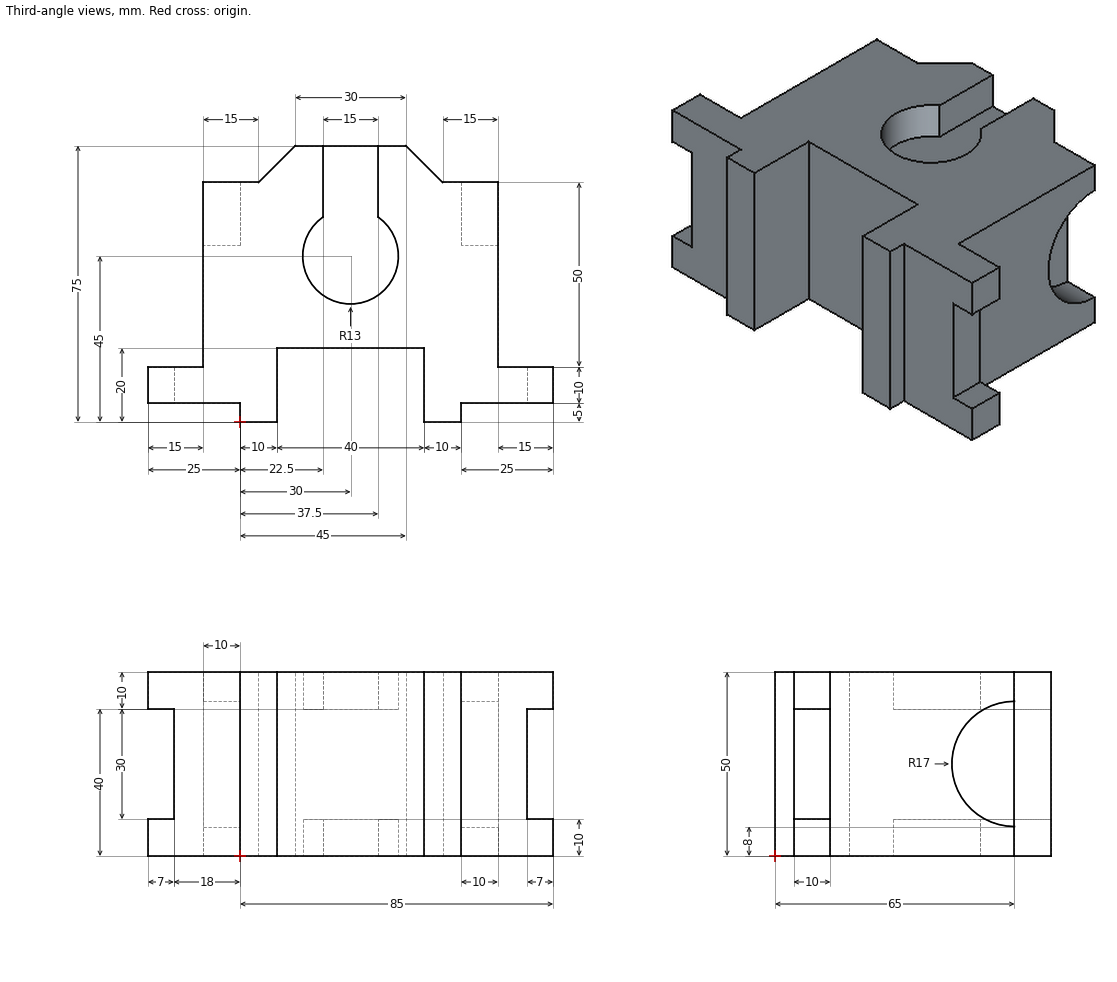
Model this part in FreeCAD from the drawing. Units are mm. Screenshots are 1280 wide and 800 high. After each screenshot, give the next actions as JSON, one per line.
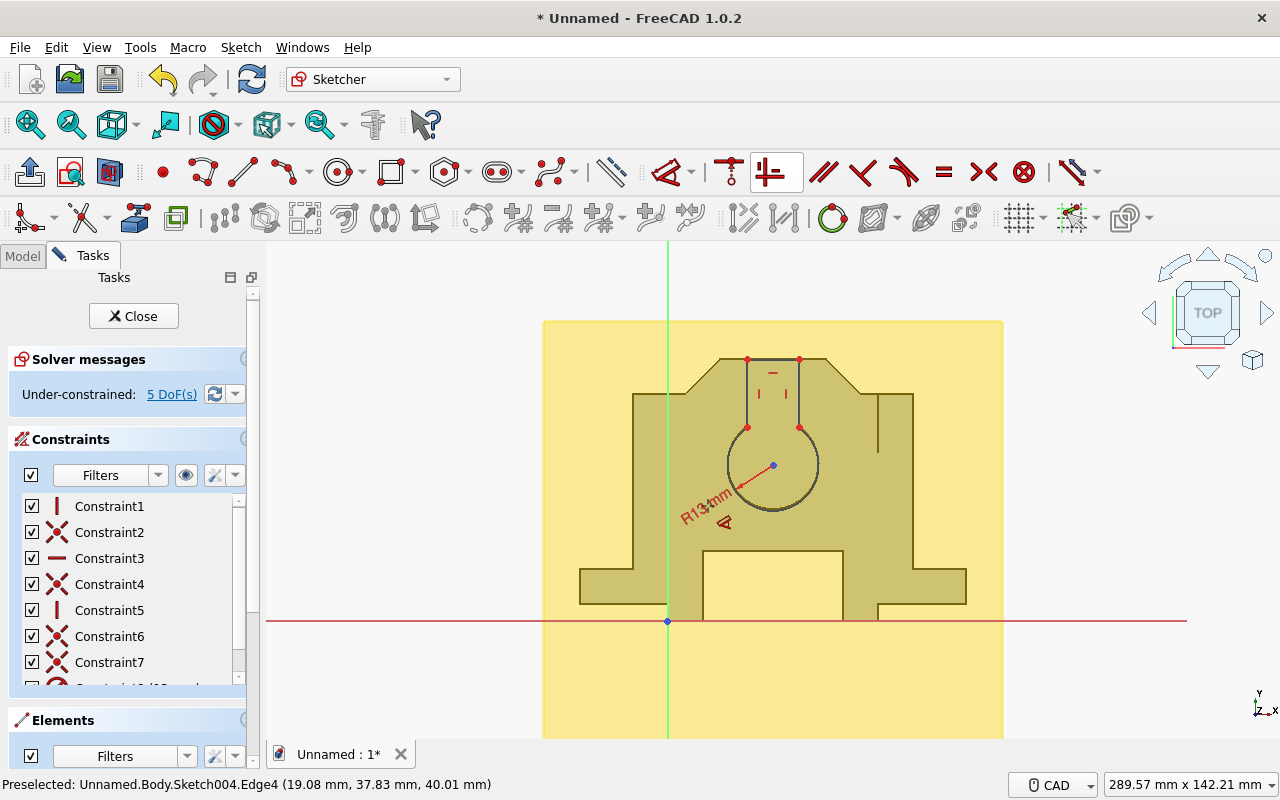
{"action": "left_click", "coordinate": [783, 360]}
{"action": "left_click", "coordinate": [773, 326]}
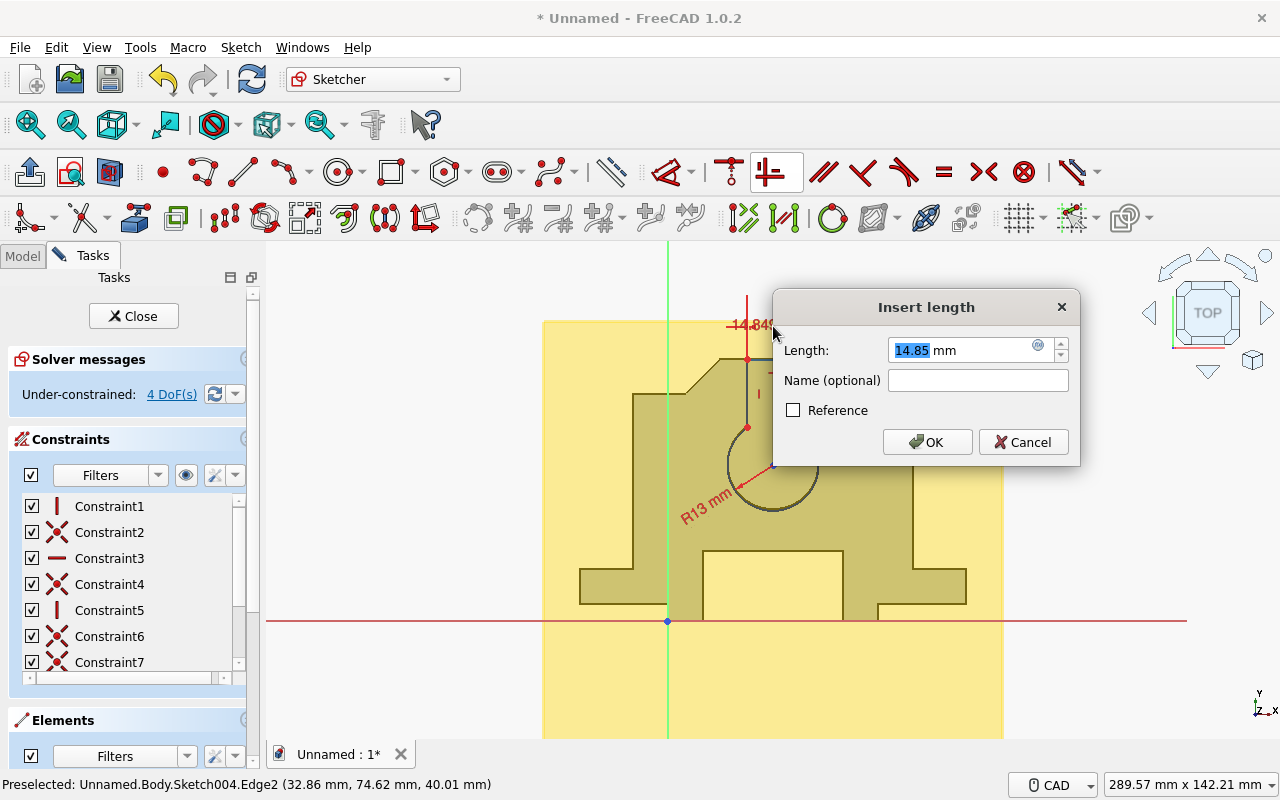
{"action": "type", "text": "15"}
{"action": "key", "text": "Return"}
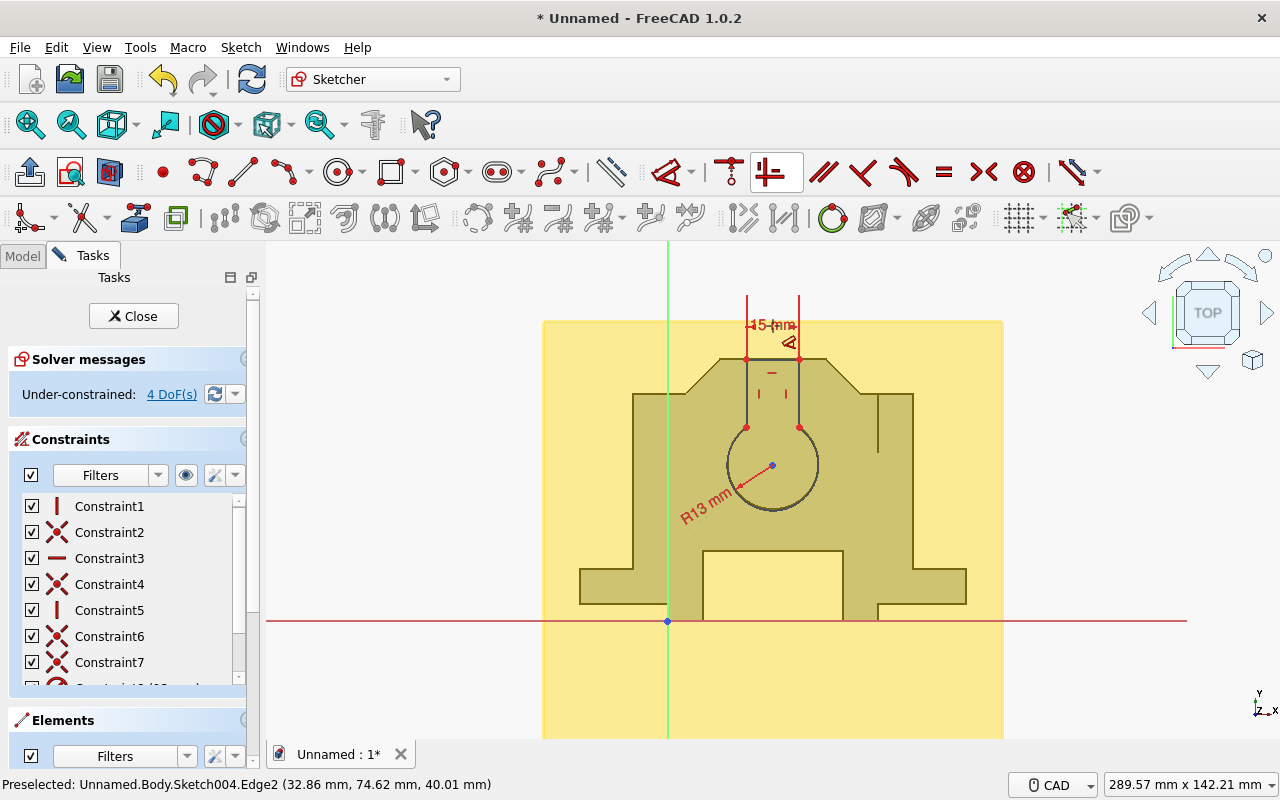
{"action": "left_click", "coordinate": [799, 360]}
{"action": "left_click", "coordinate": [634, 491]}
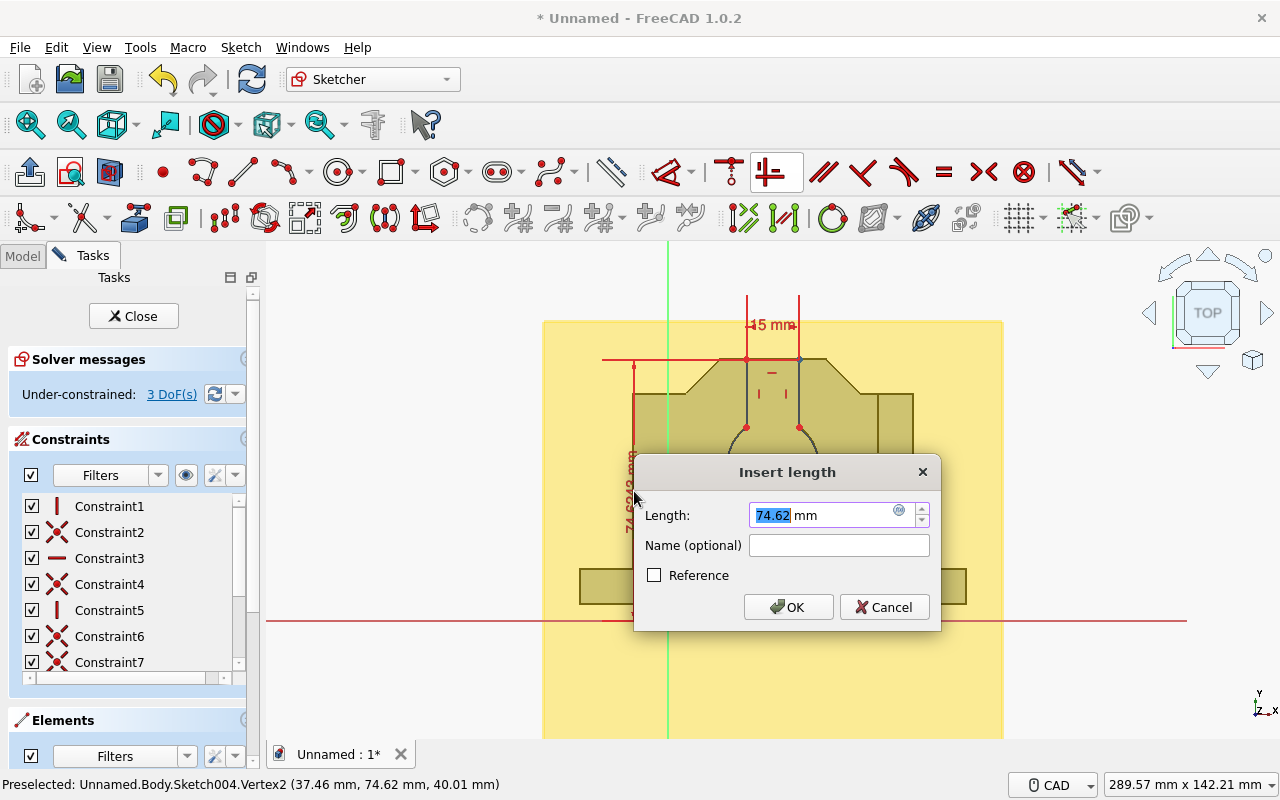
{"action": "type", "text": "75"}
{"action": "key", "text": "Return"}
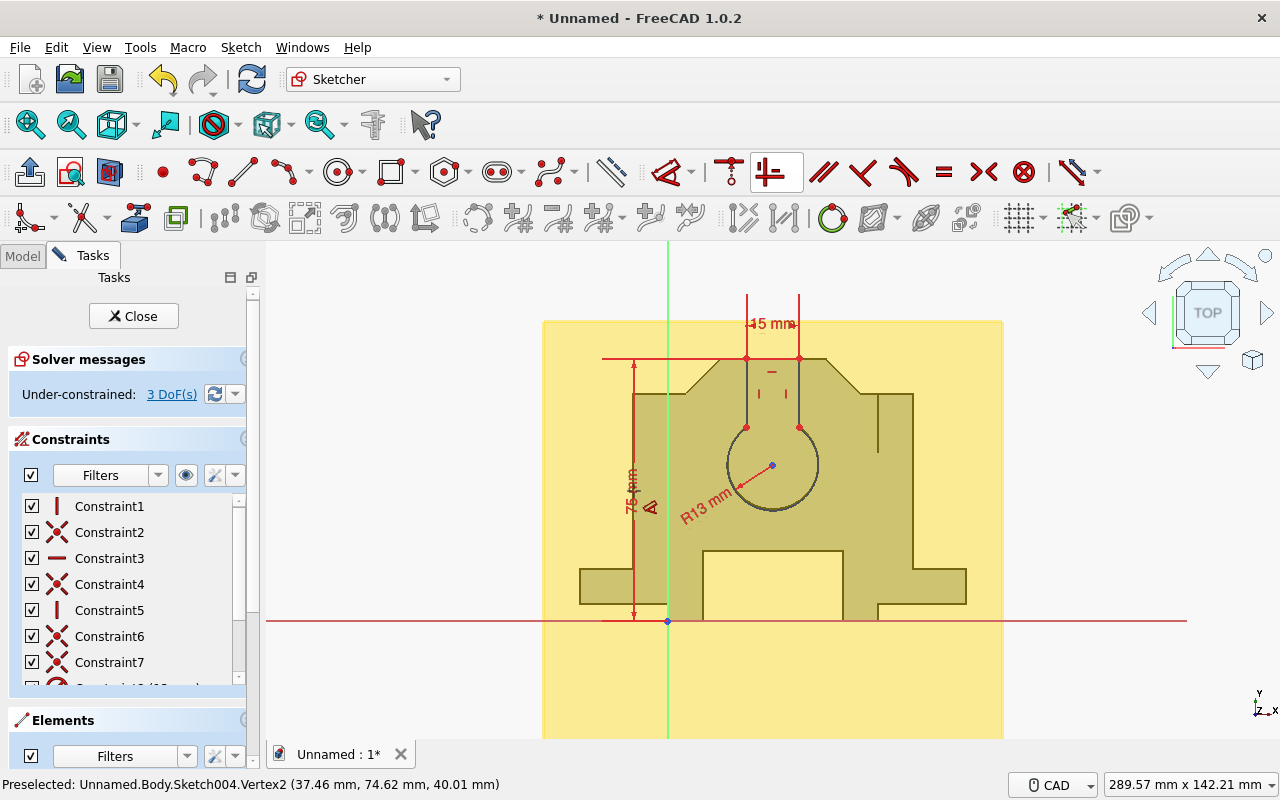
{"action": "left_click", "coordinate": [773, 465]}
{"action": "left_click", "coordinate": [720, 655]}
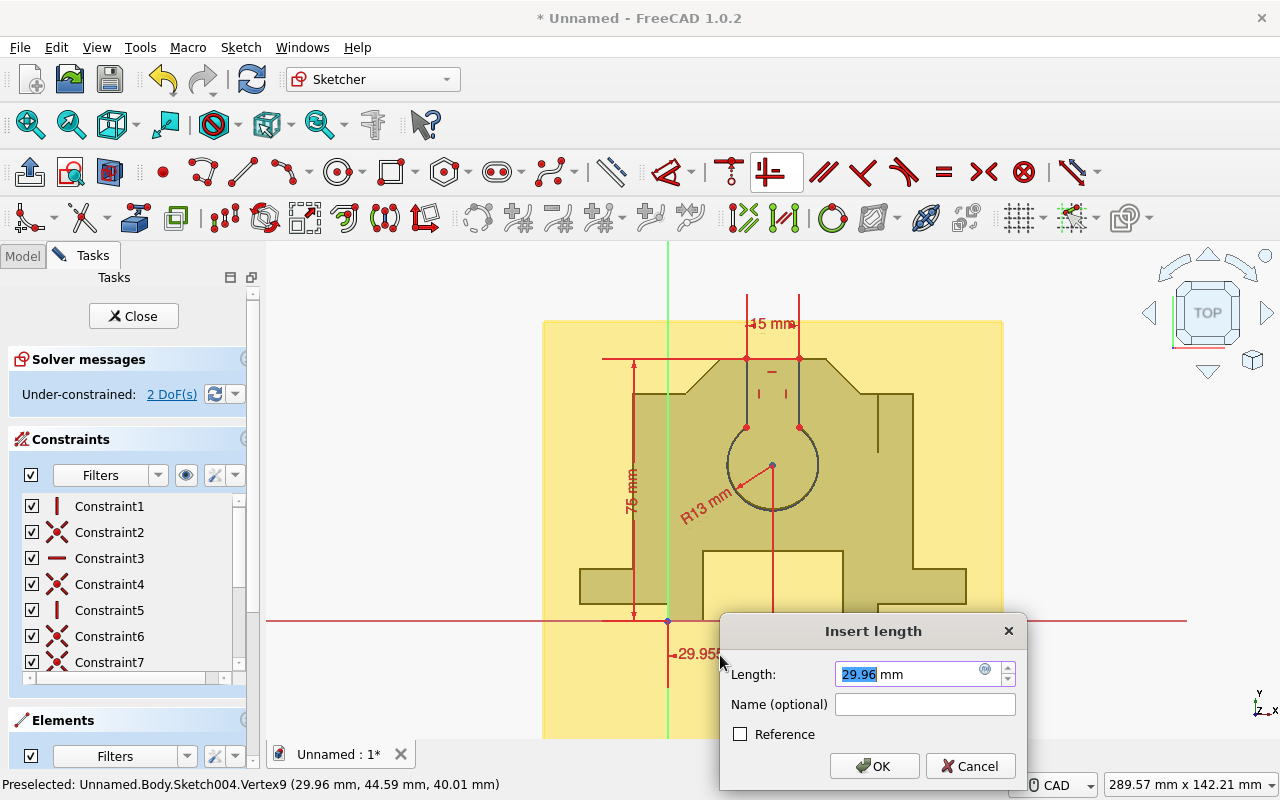
{"action": "type", "text": "30"}
{"action": "key", "text": "Return"}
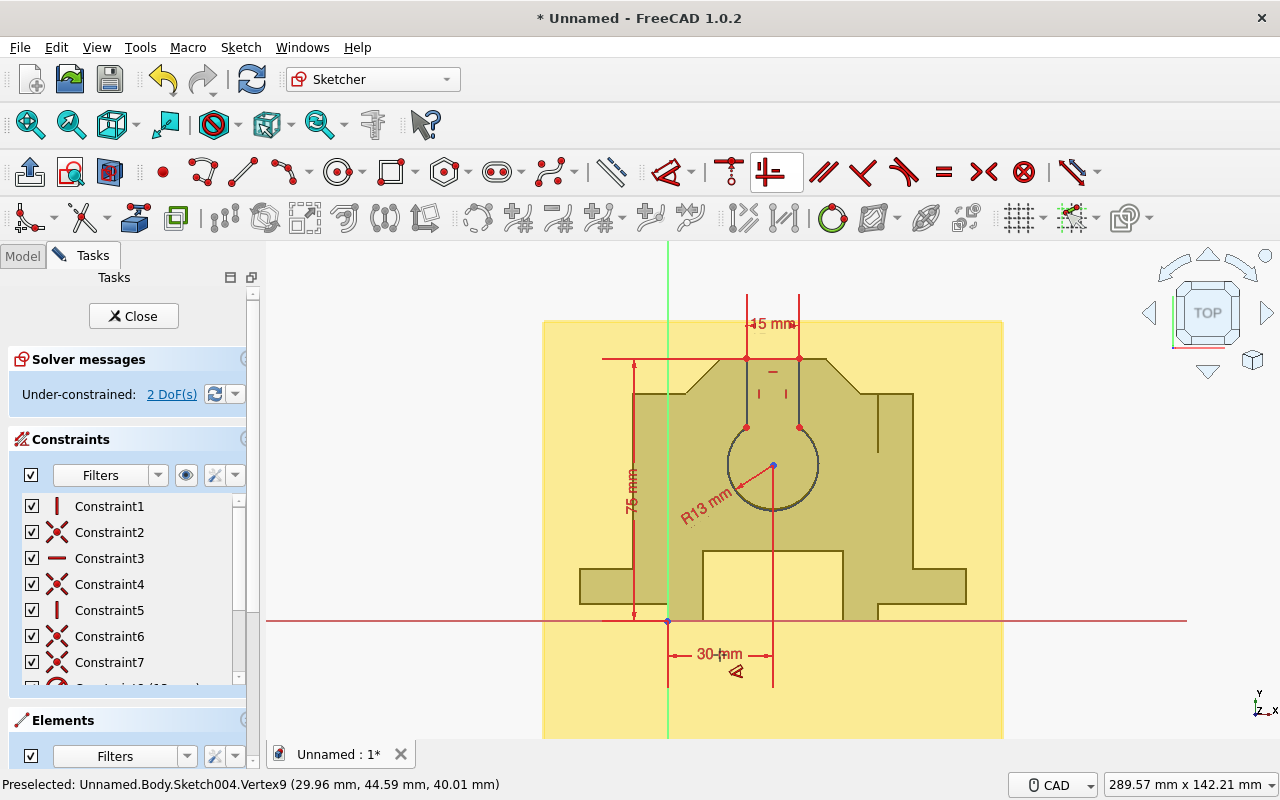
{"action": "left_click", "coordinate": [773, 465]}
{"action": "left_click", "coordinate": [634, 543]}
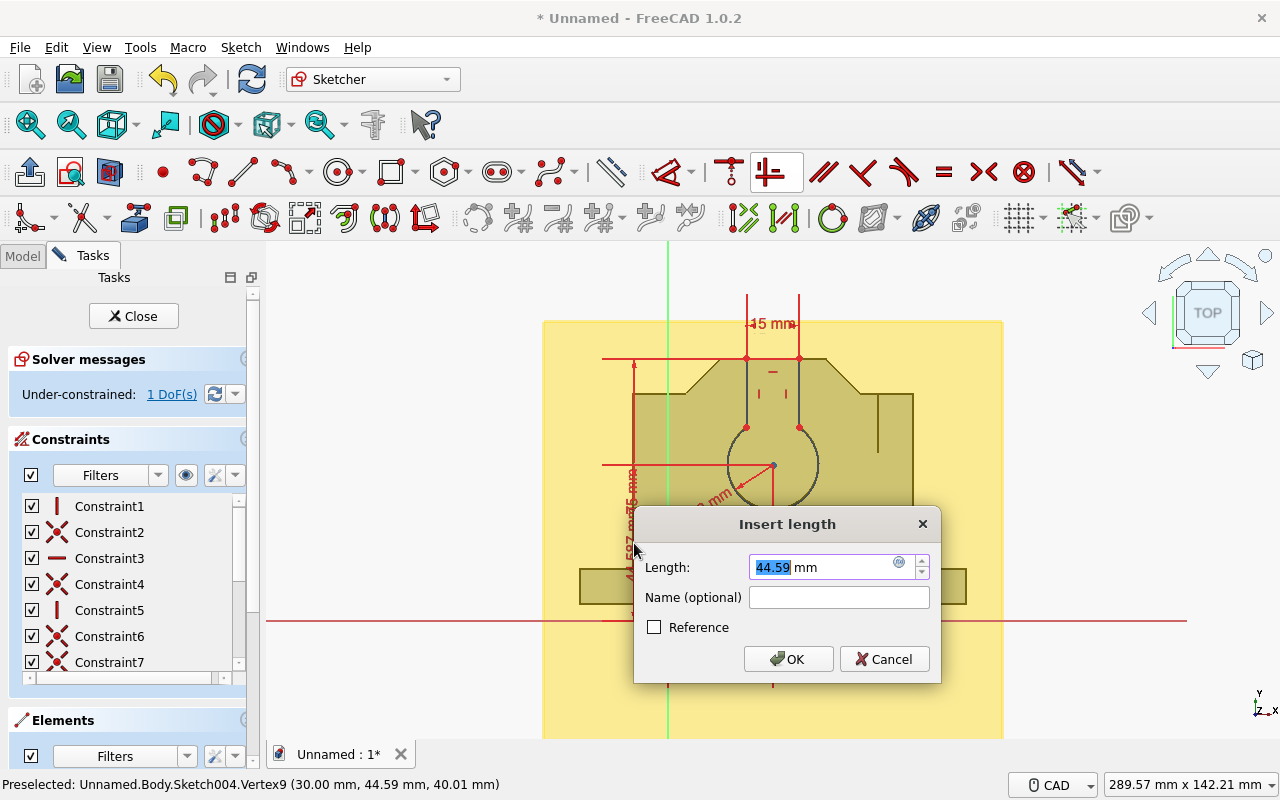
{"action": "type", "text": "45"}
{"action": "key", "text": "Return"}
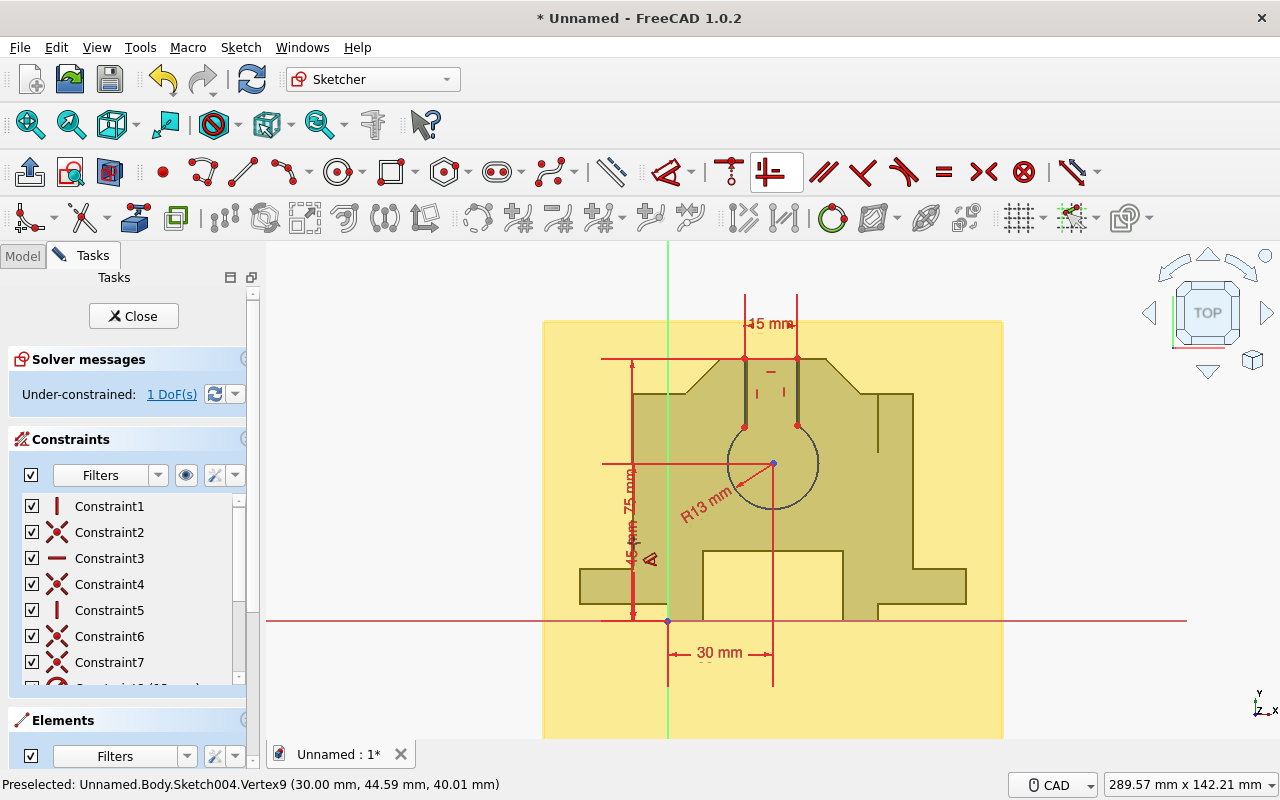
{"action": "left_click", "coordinate": [797, 425]}
{"action": "left_click", "coordinate": [703, 391]}